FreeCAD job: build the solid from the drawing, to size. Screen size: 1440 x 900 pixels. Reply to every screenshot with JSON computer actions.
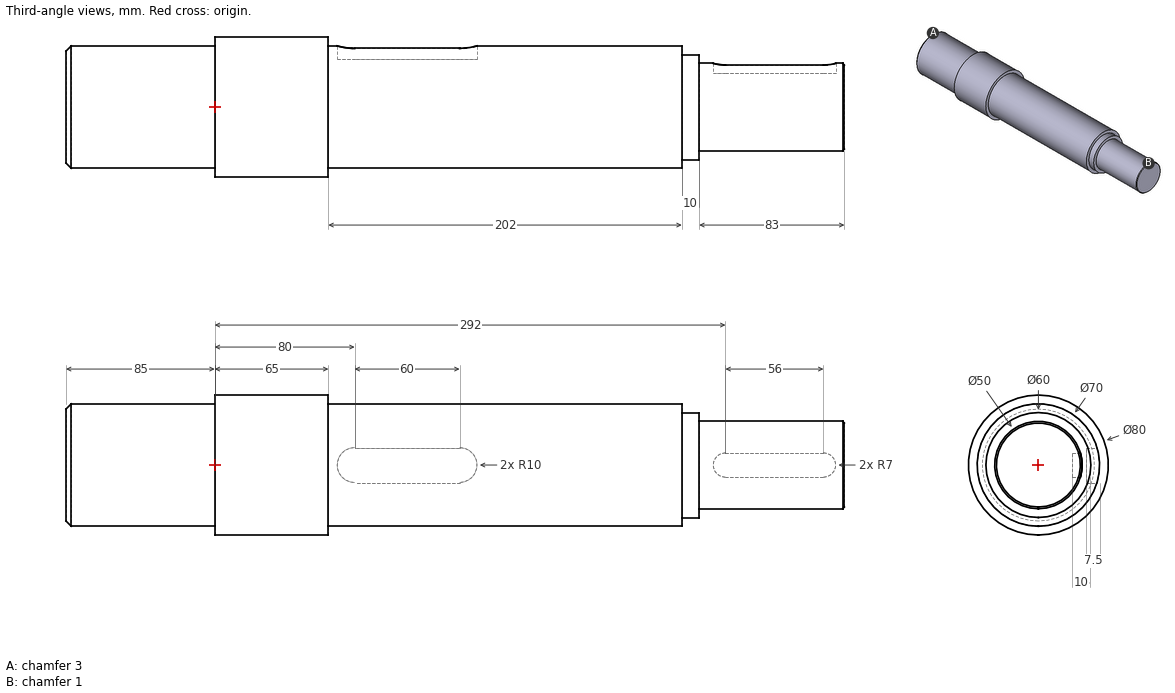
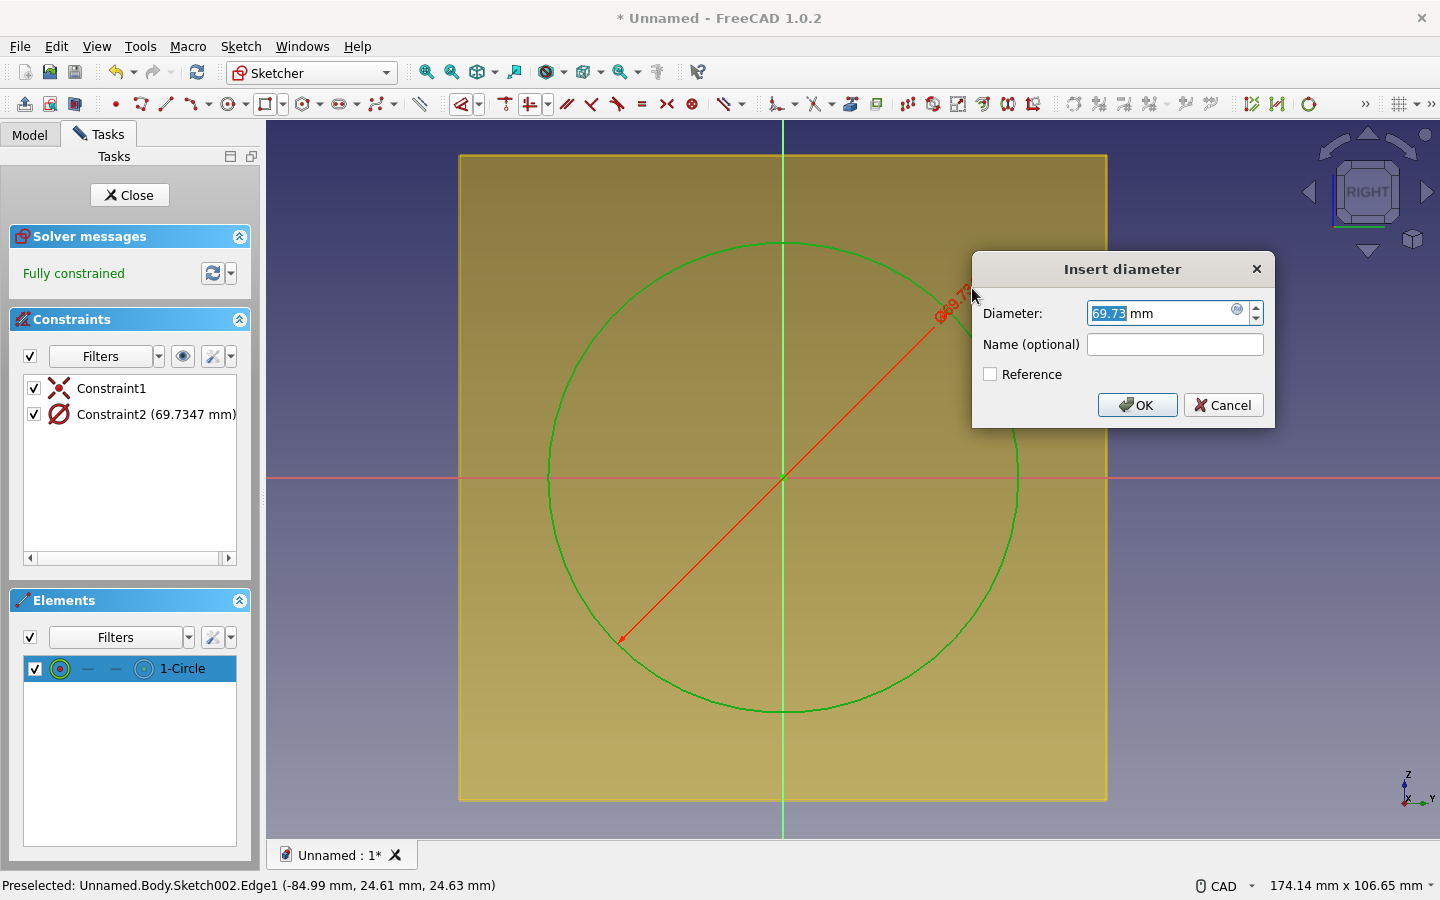
{"action": "type", "text": "70"}
{"action": "key", "text": "Return"}
{"action": "key", "text": "Escape"}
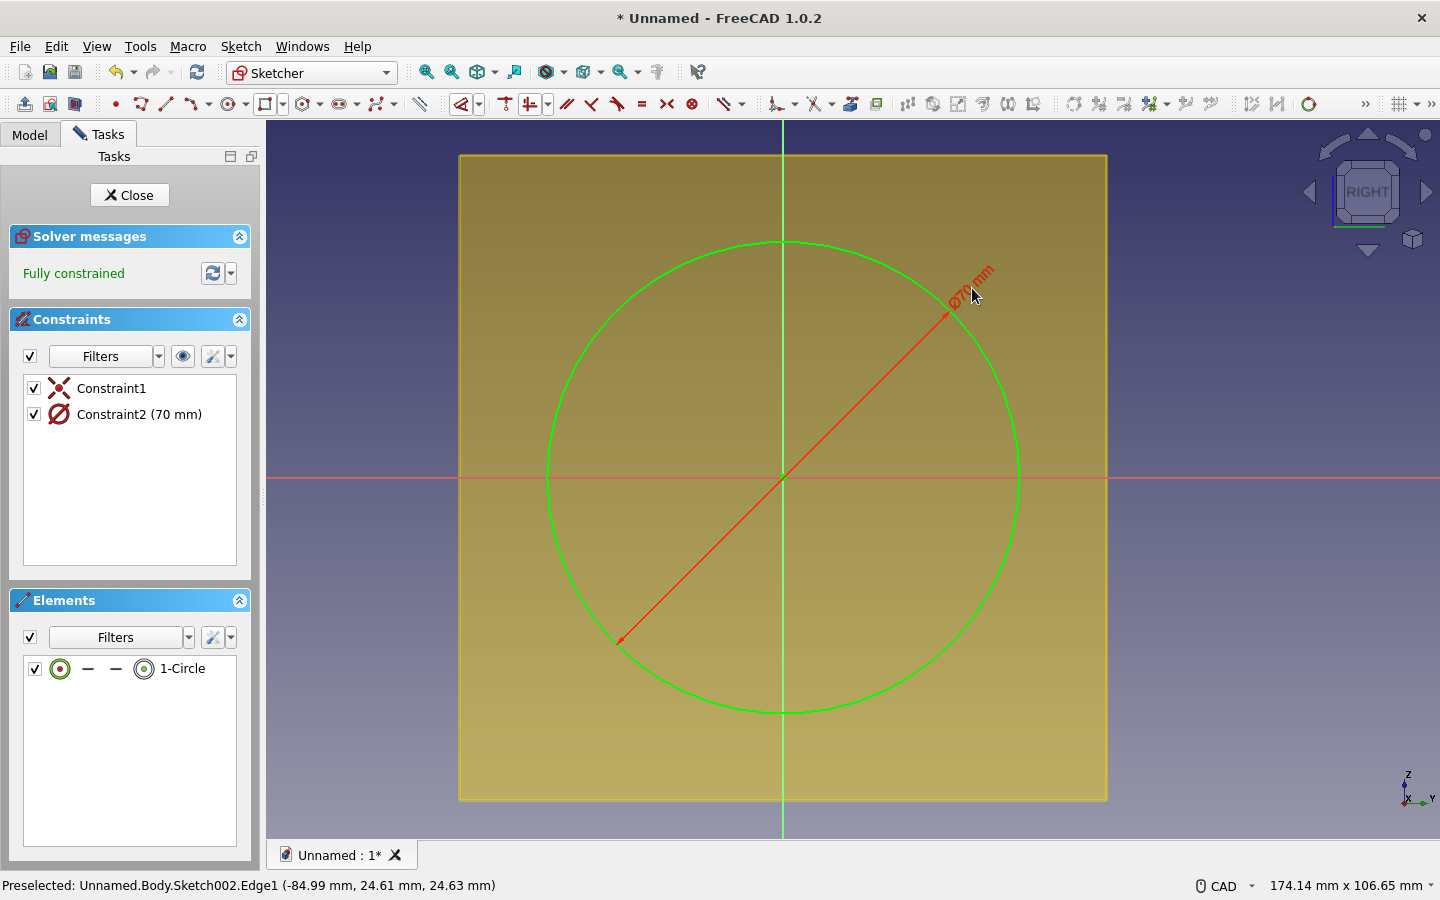
{"action": "left_click", "coordinate": [130, 195]}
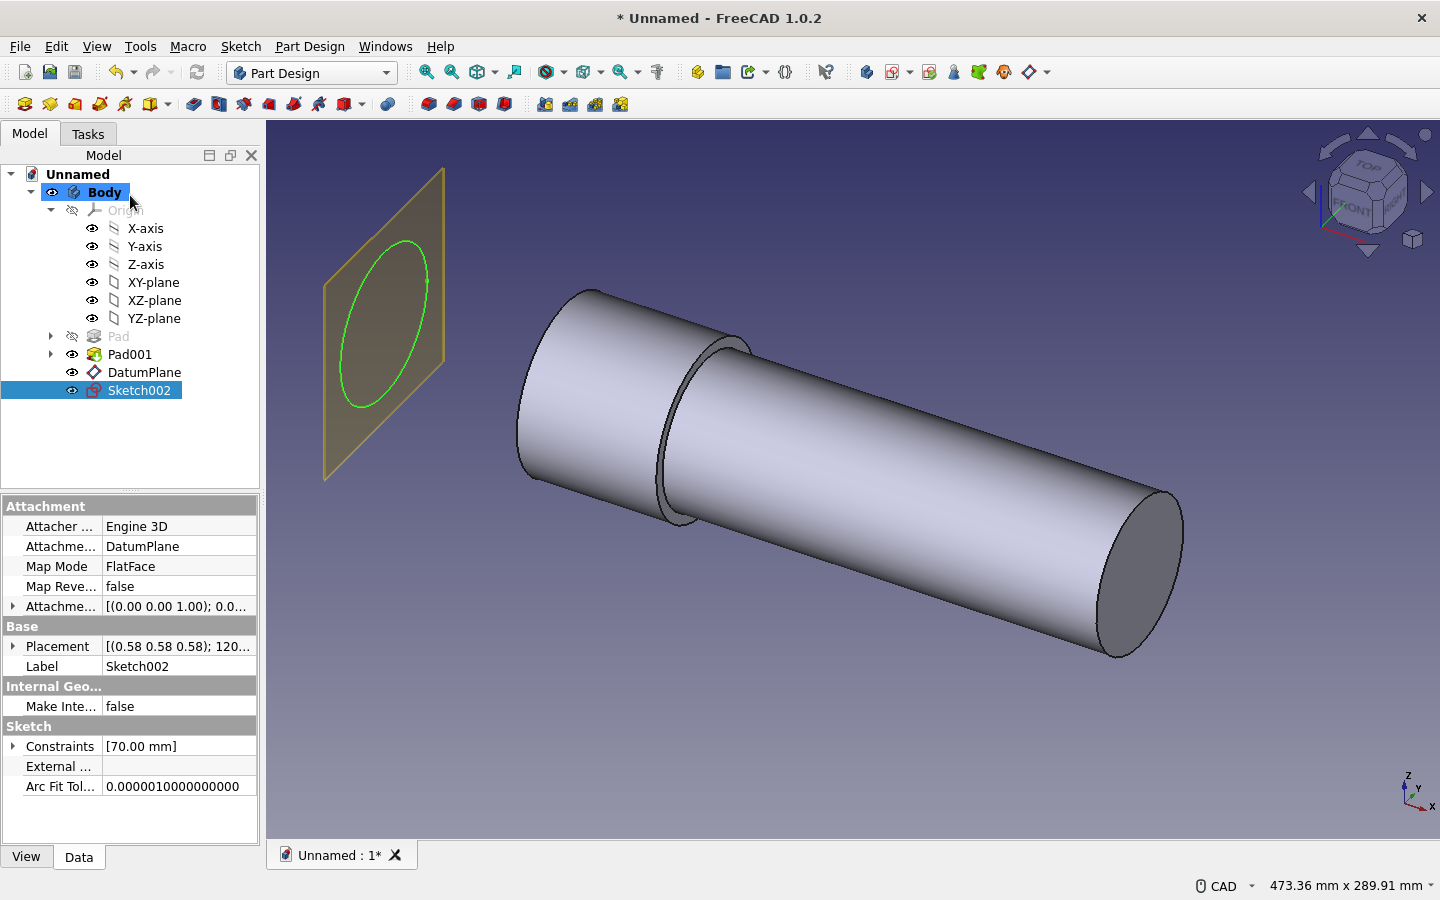
{"action": "left_click", "coordinate": [25, 104]}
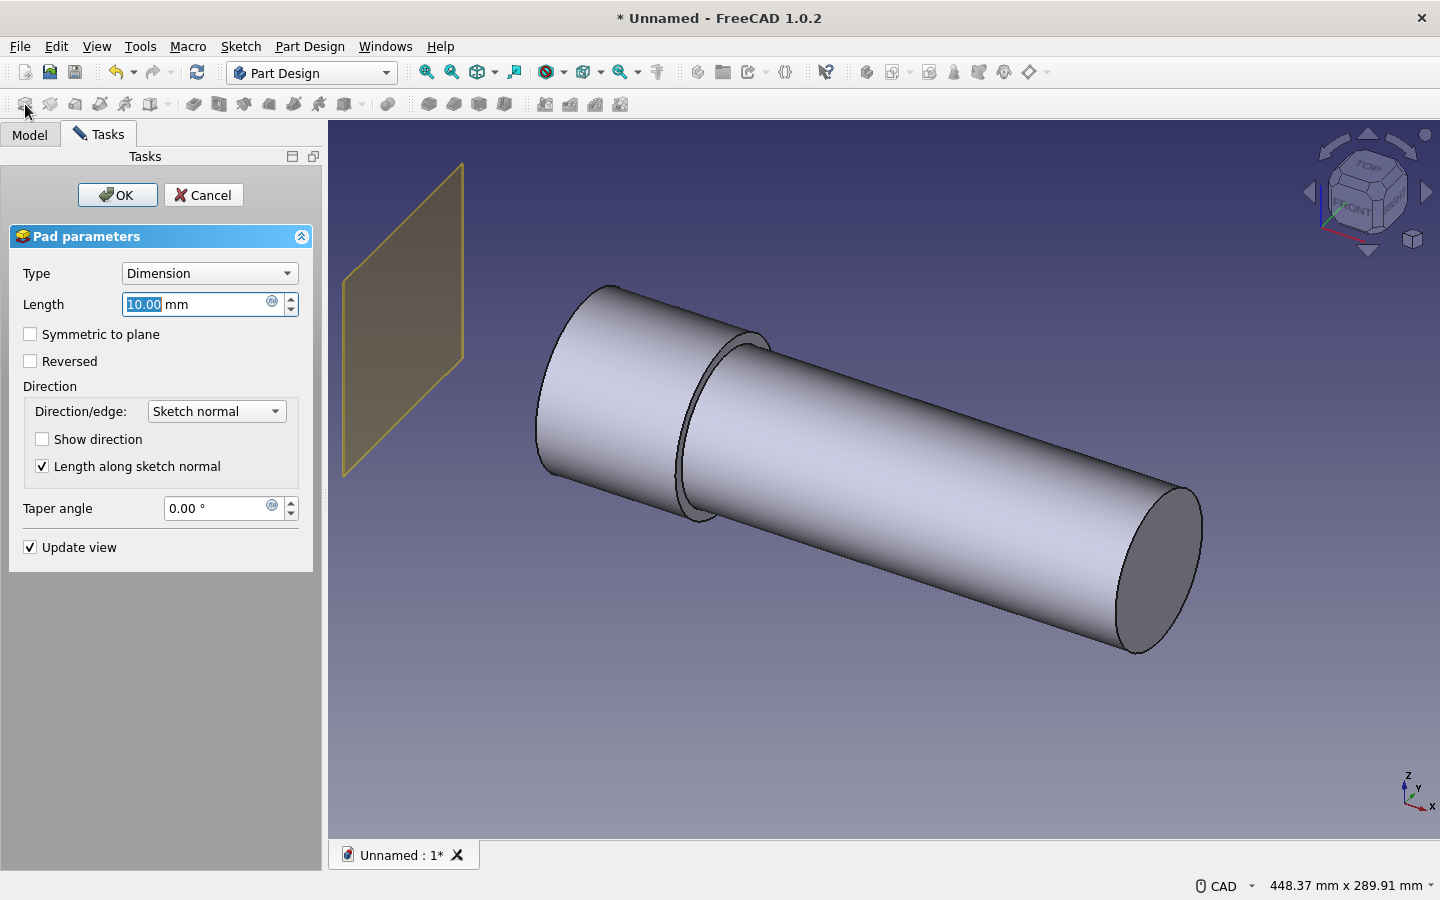
{"action": "type", "text": "85"}
{"action": "key", "text": "Tab"}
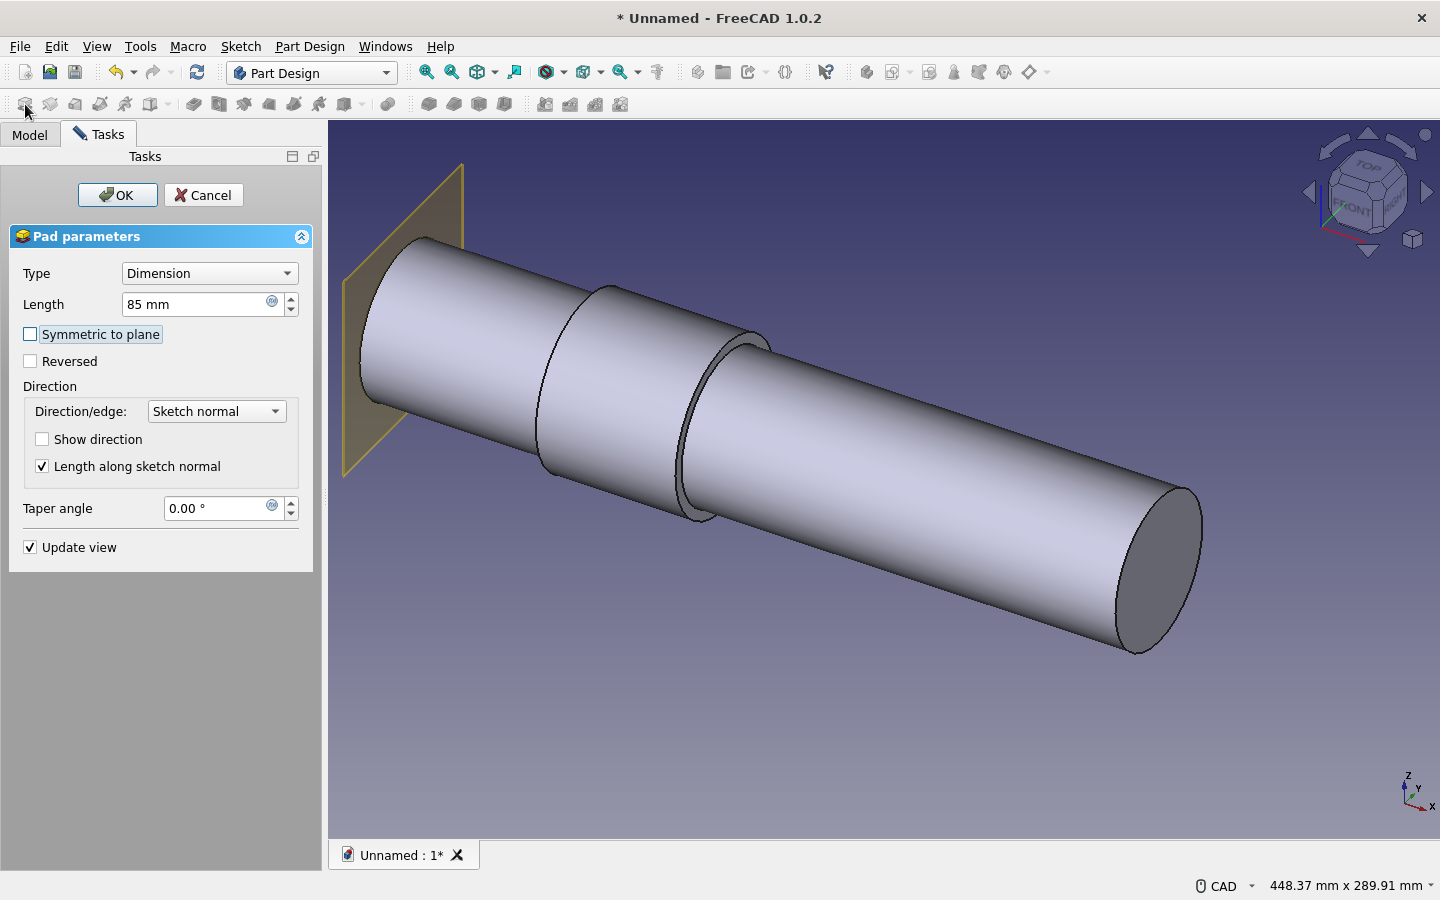
{"action": "left_click", "coordinate": [118, 195]}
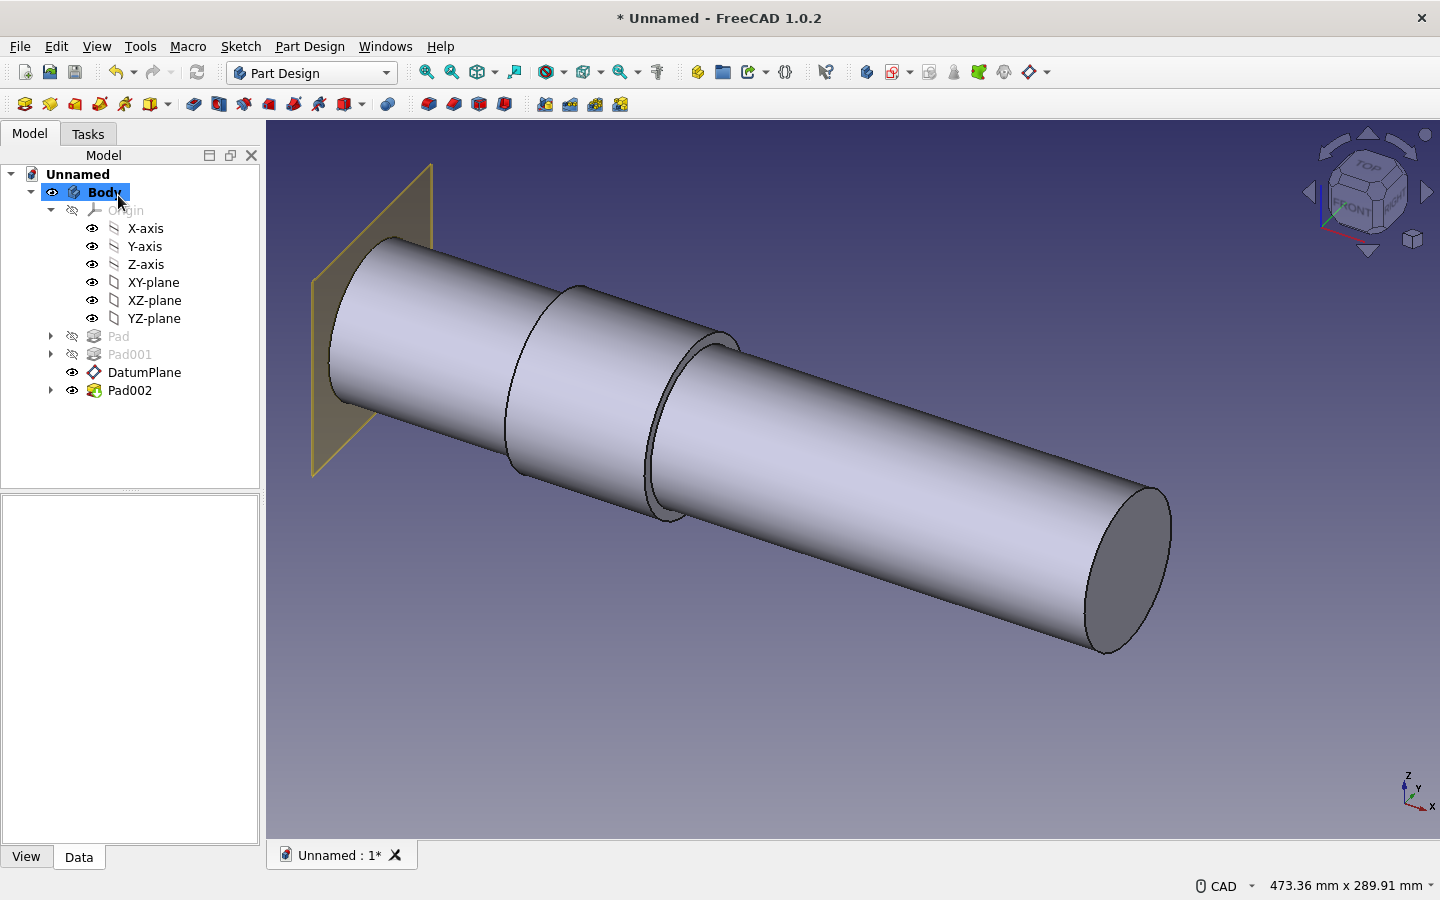
{"action": "left_click", "coordinate": [117, 372]}
{"action": "key", "text": "space"}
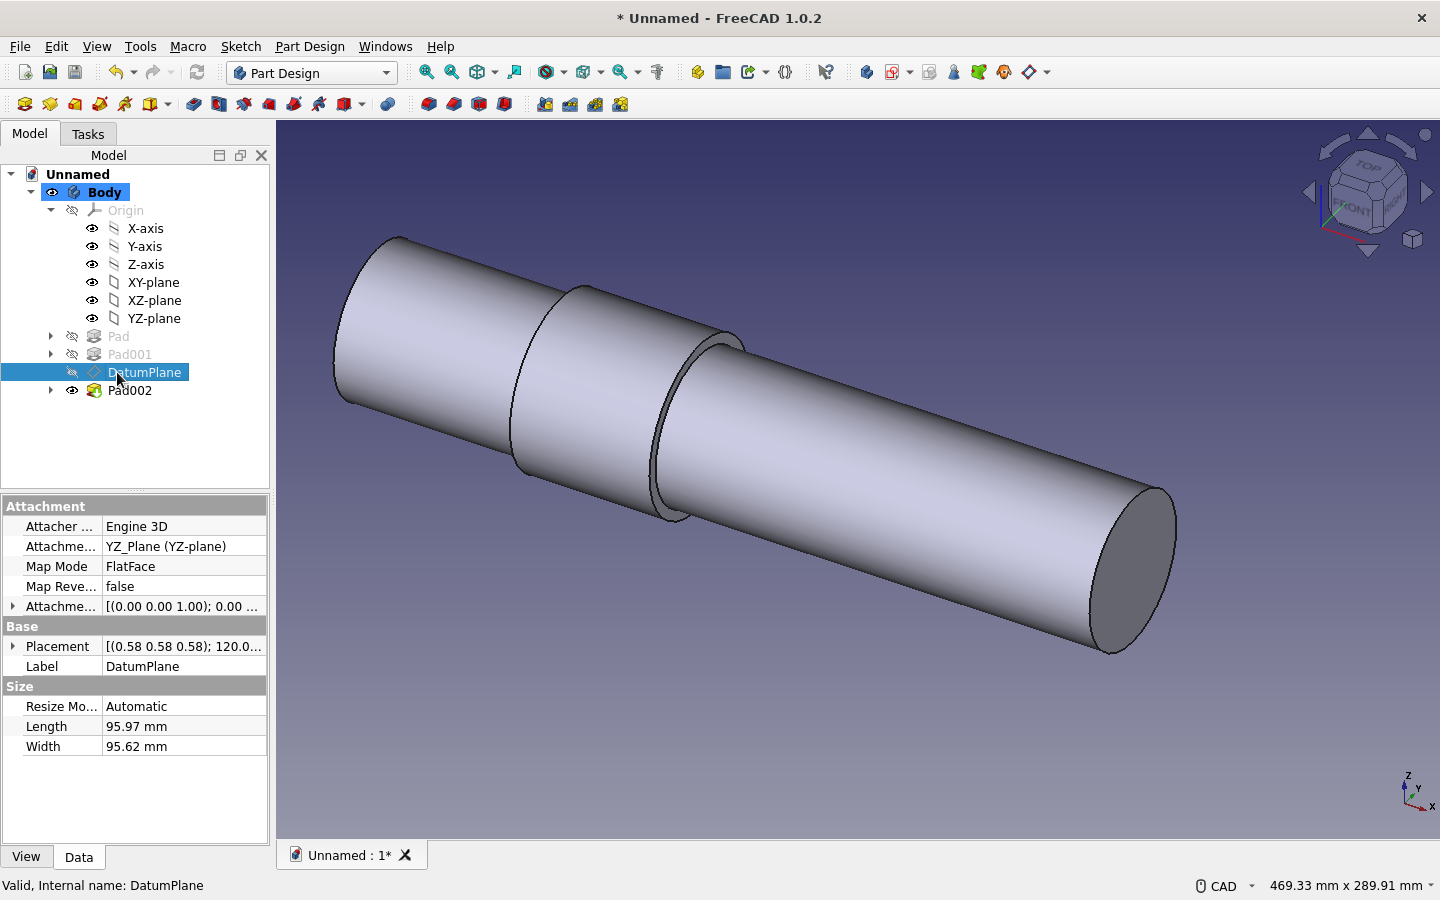
{"action": "key", "text": "0"}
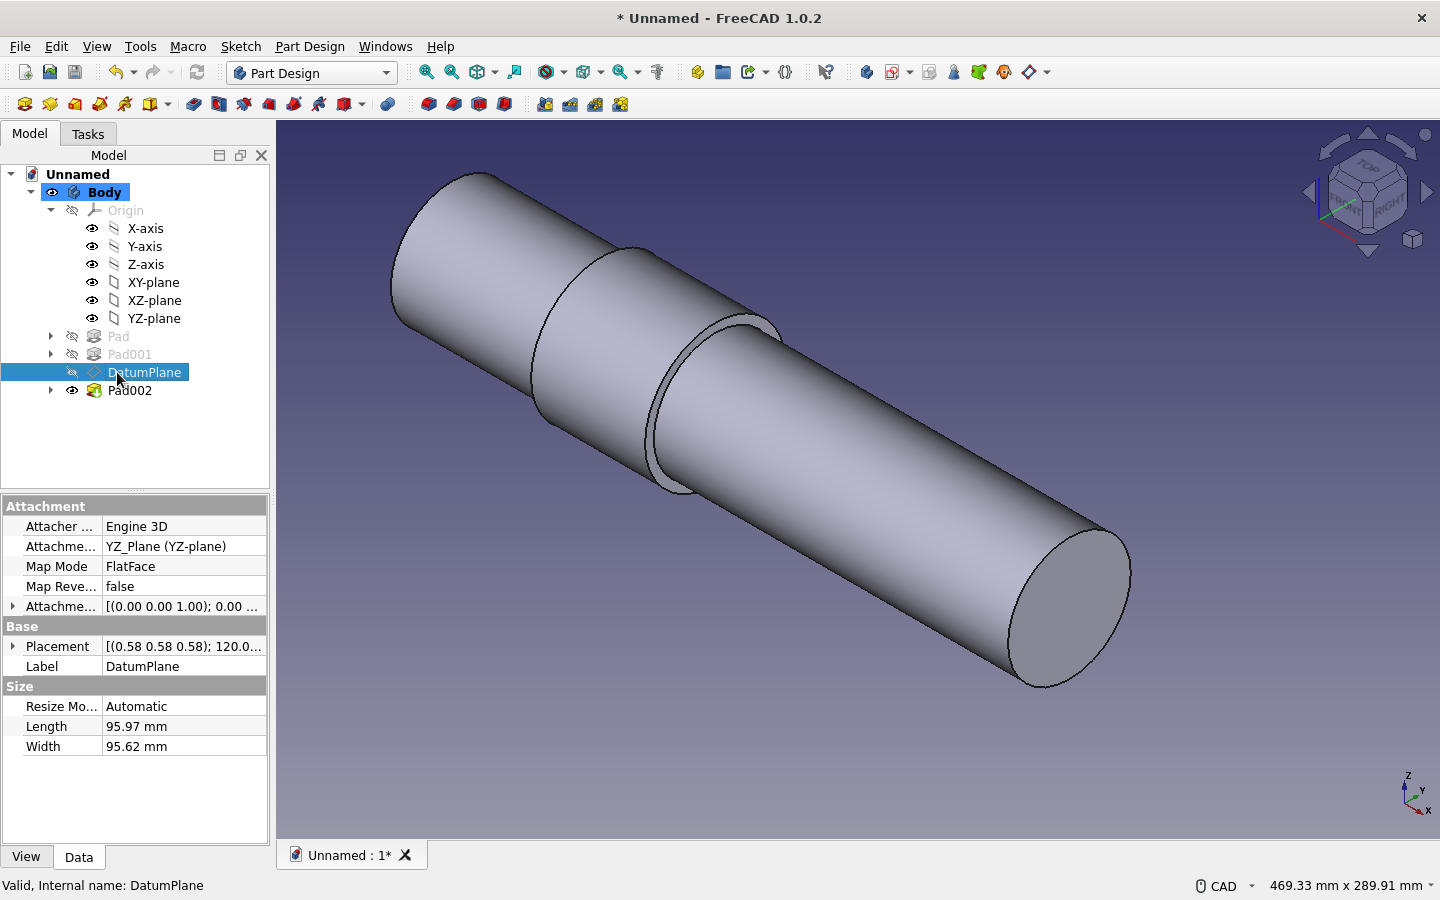
{"action": "key", "text": "2"}